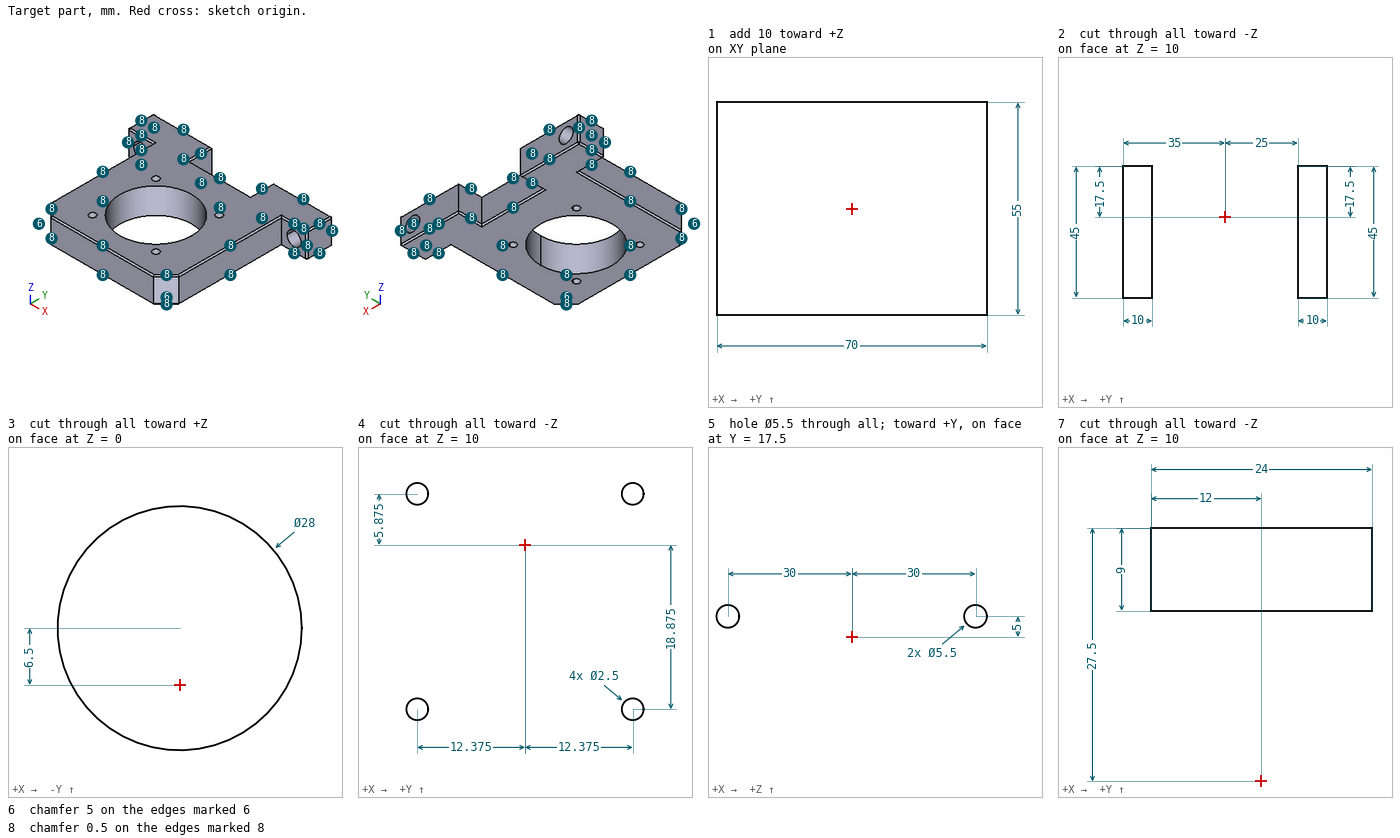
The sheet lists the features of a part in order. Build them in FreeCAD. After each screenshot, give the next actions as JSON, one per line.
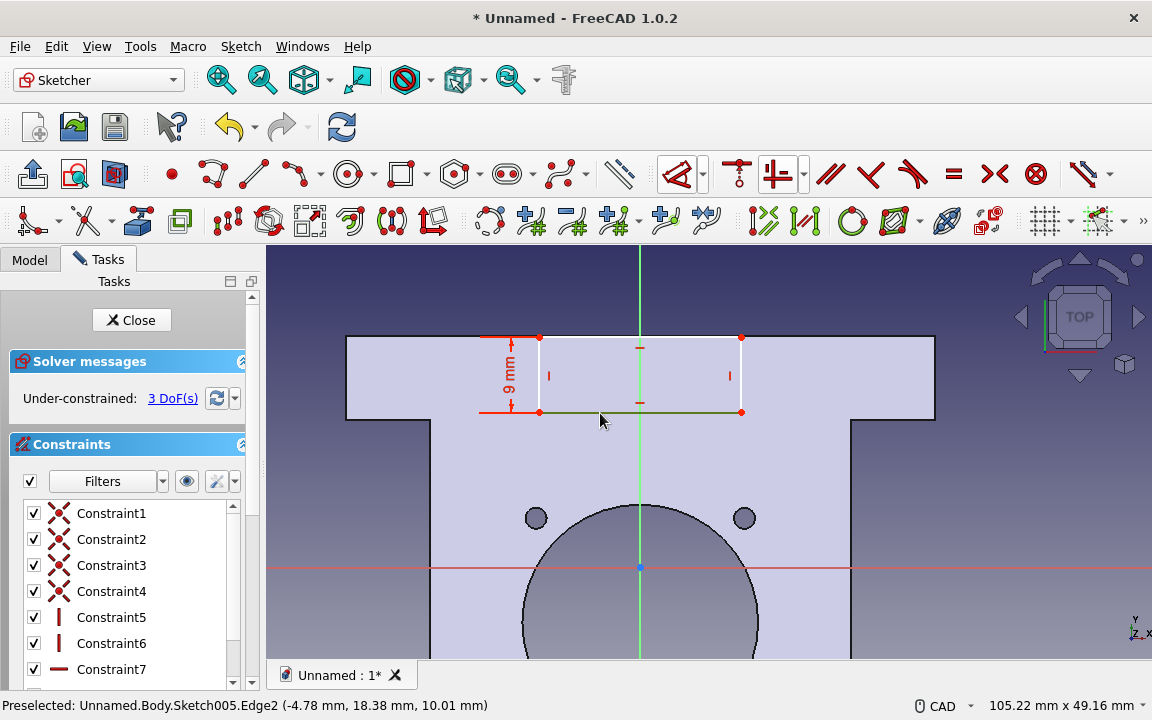
{"action": "key", "text": "l"}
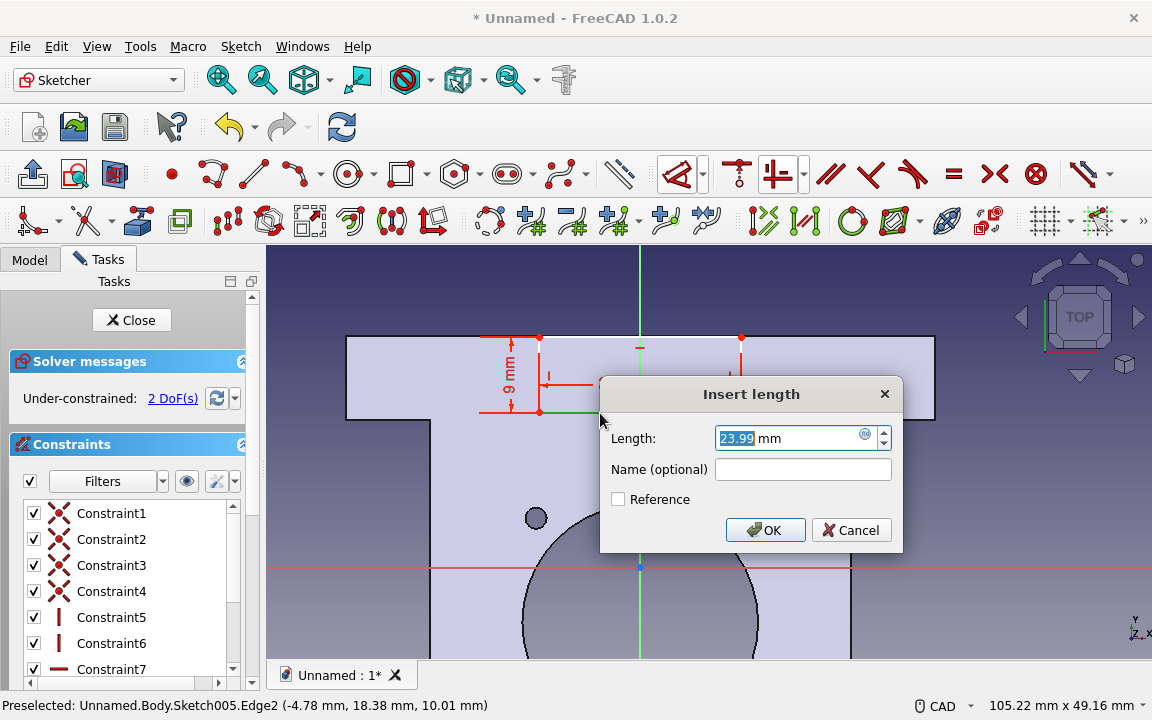
{"action": "type", "text": "24"}
{"action": "key", "text": "Return"}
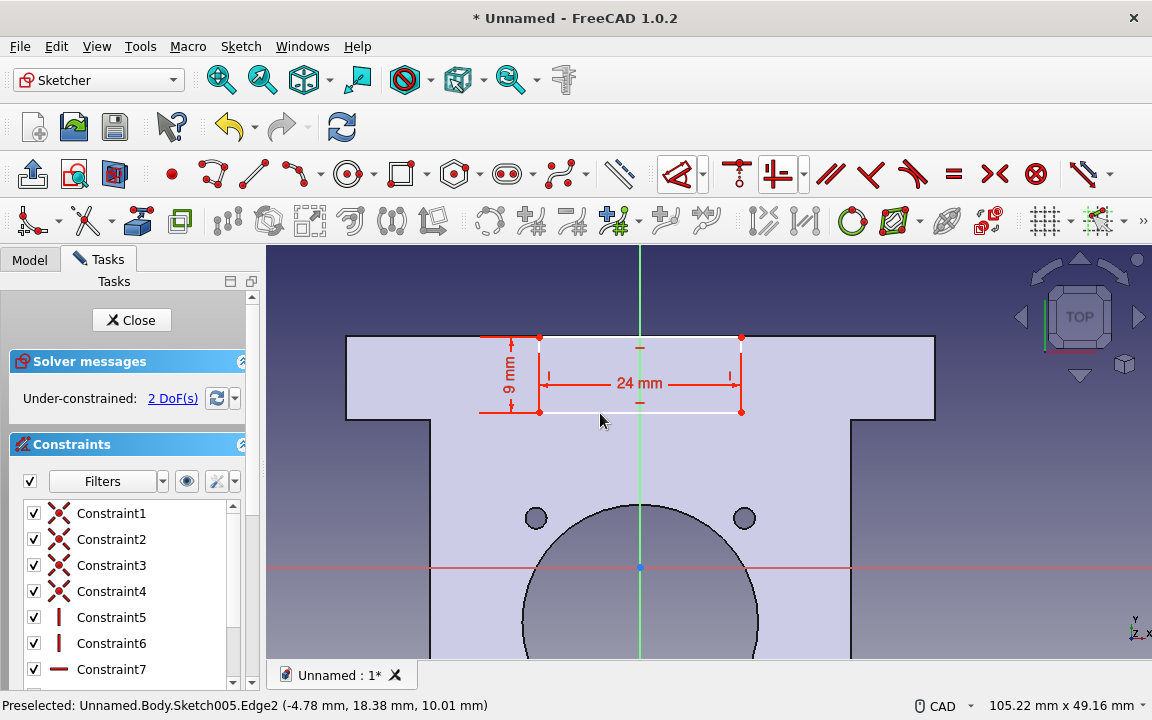
{"action": "left_click", "coordinate": [539, 337]}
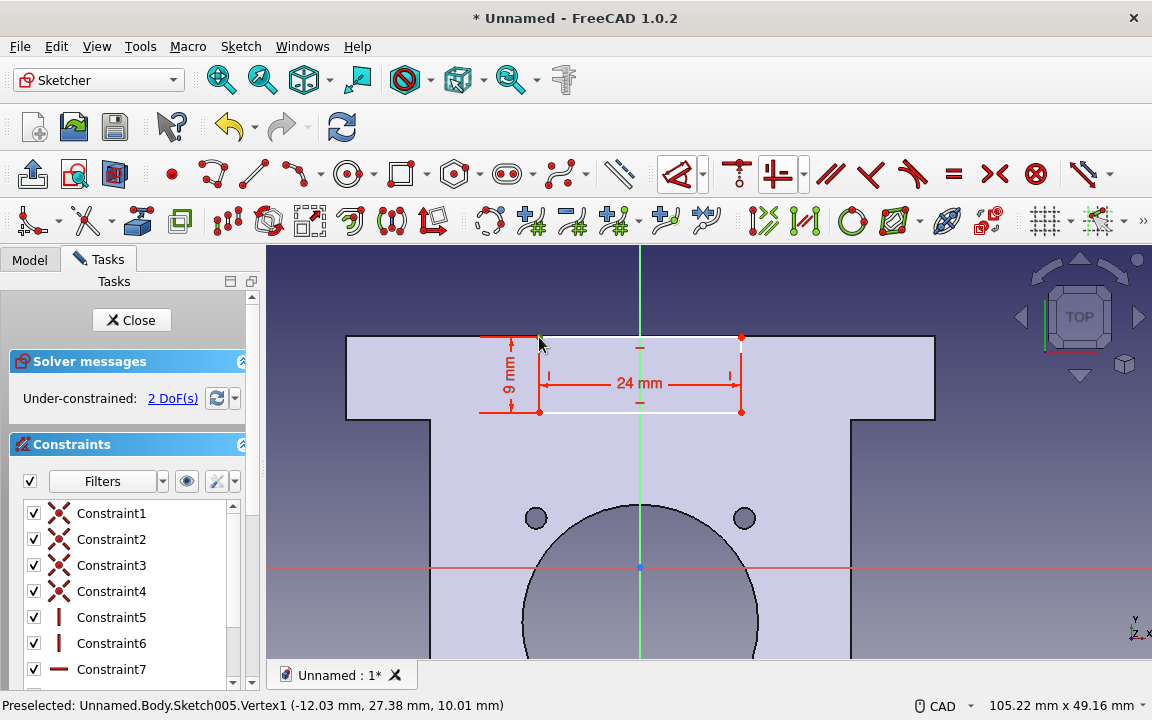
{"action": "left_click", "coordinate": [702, 174]}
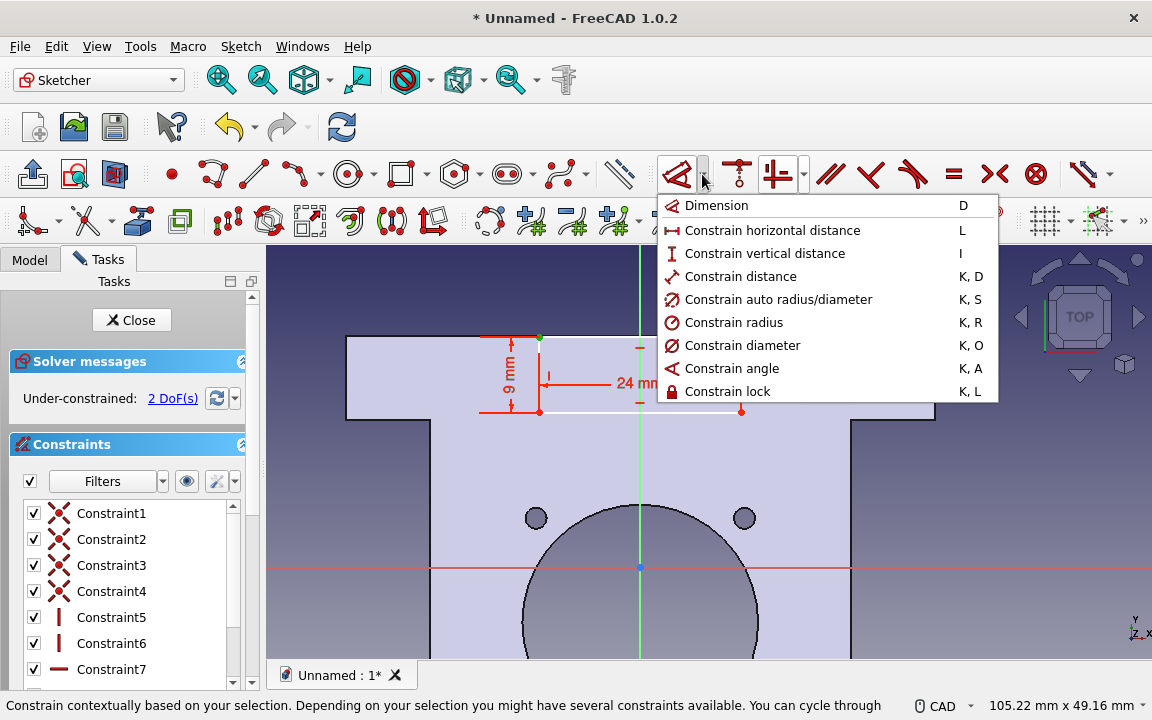
{"action": "left_click", "coordinate": [828, 230]}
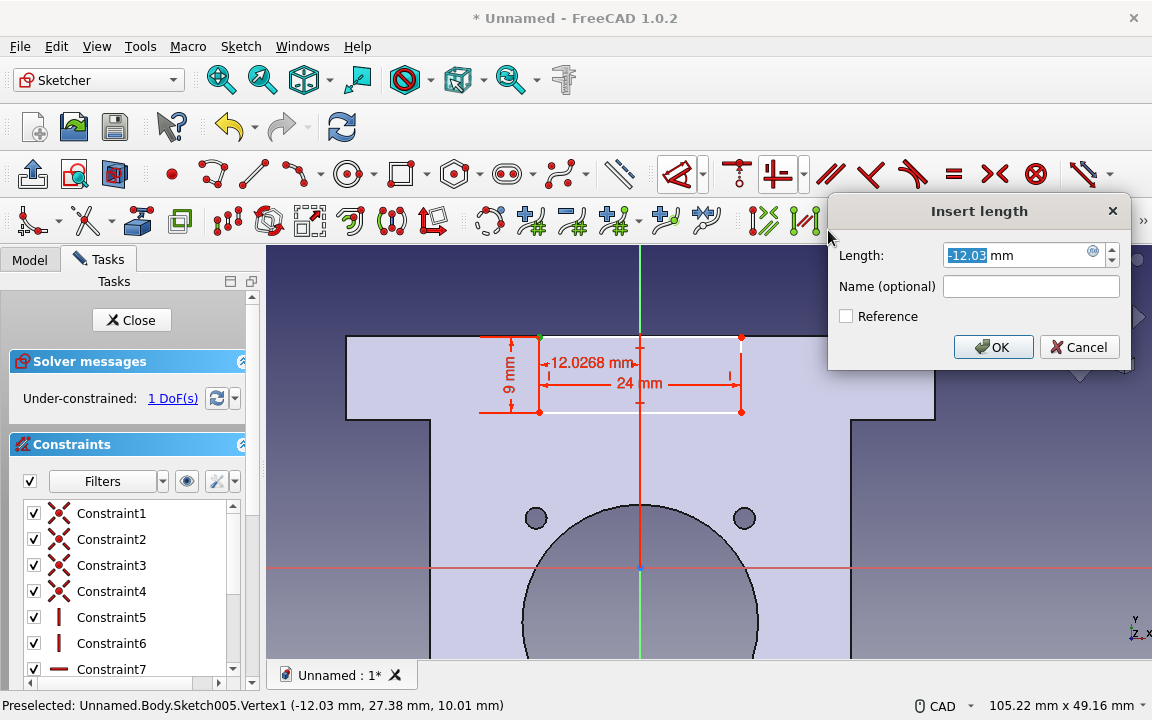
{"action": "type", "text": "-12"}
{"action": "key", "text": "Return"}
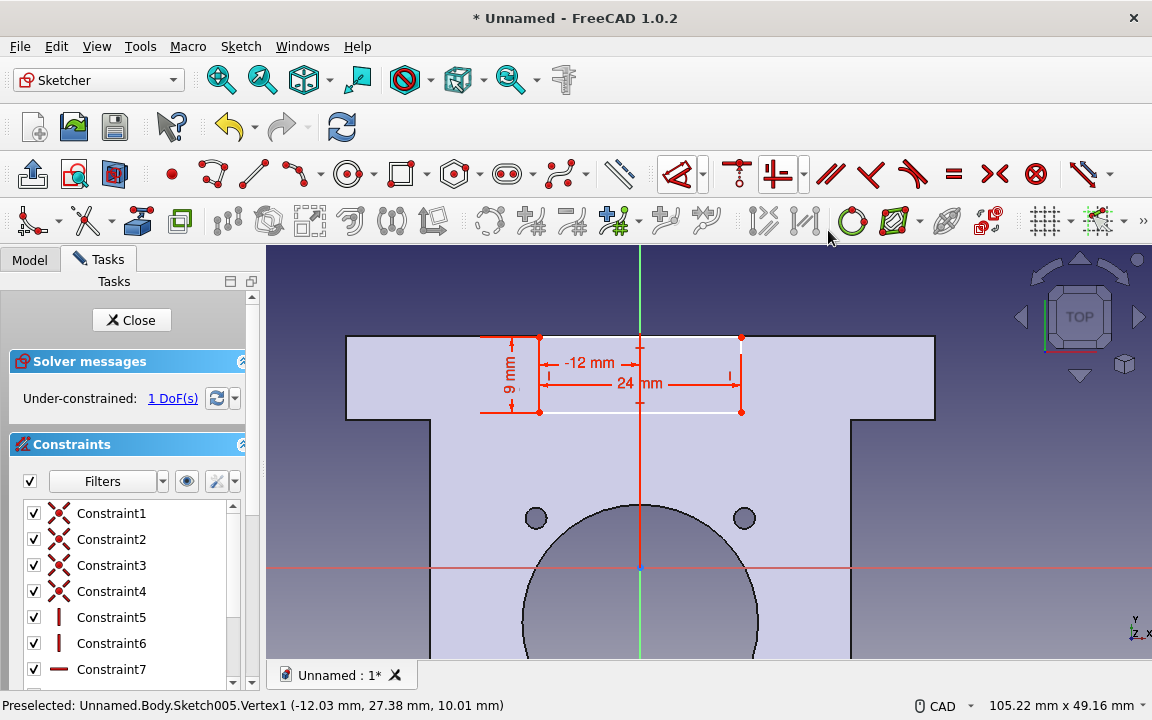
{"action": "left_click", "coordinate": [539, 337]}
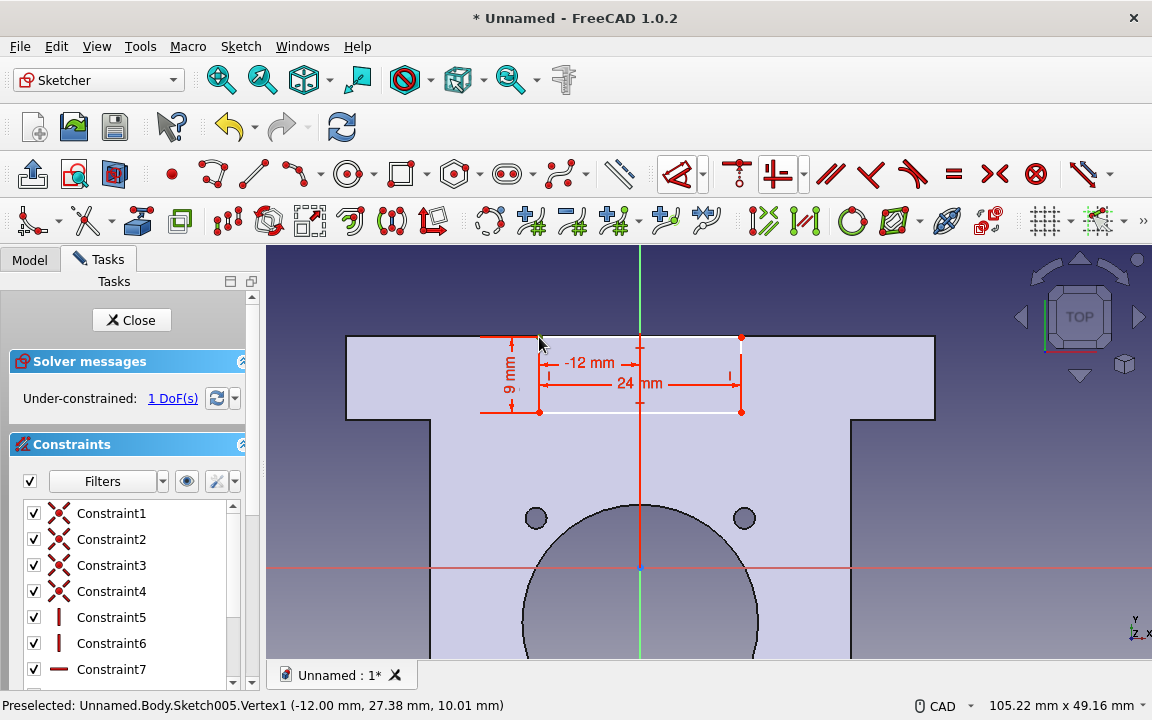
{"action": "left_click", "coordinate": [702, 174]}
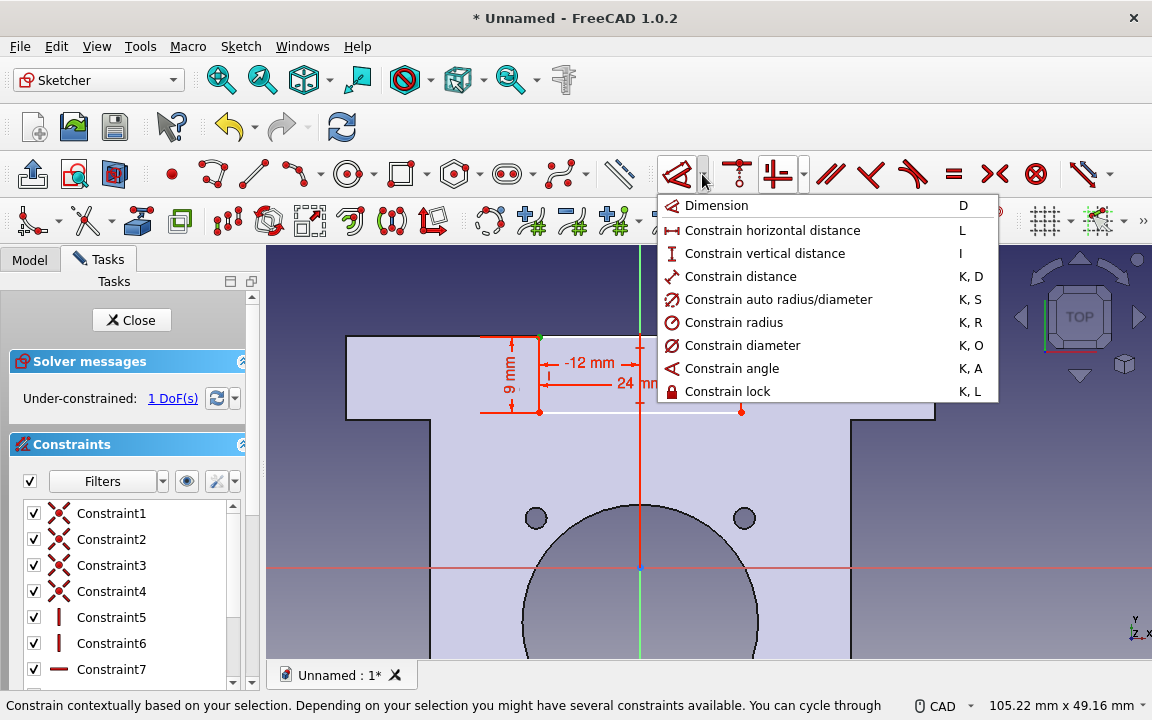
{"action": "left_click", "coordinate": [828, 254]}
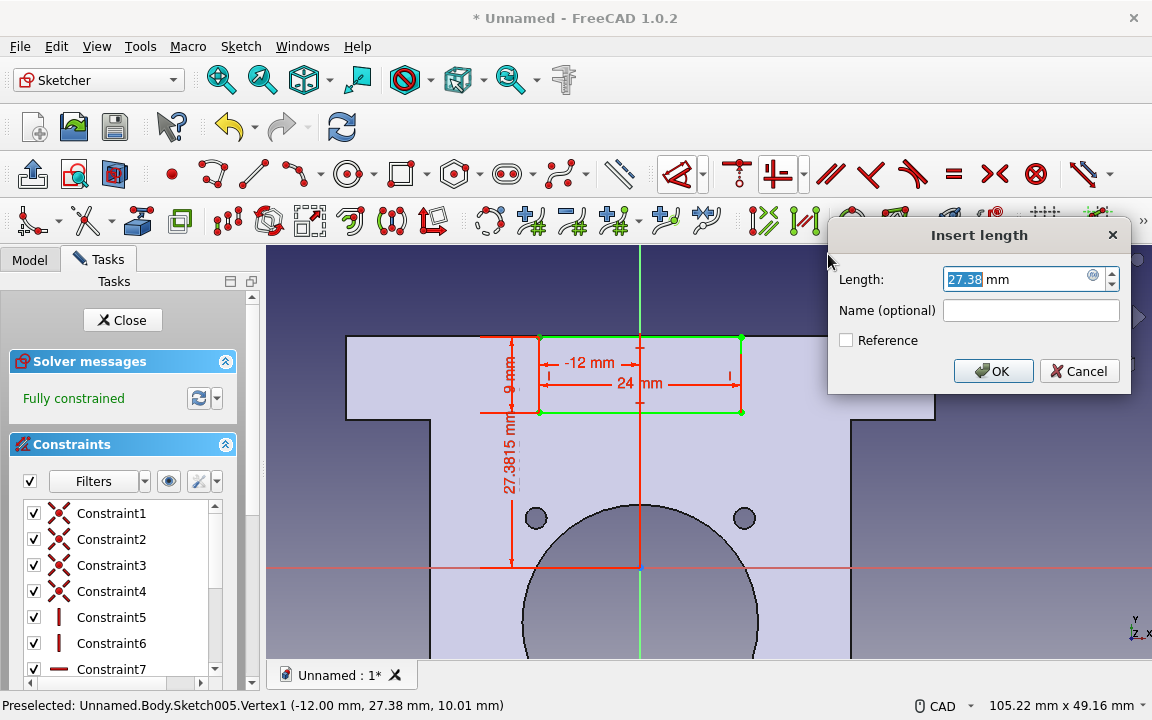
{"action": "type", "text": "27.5"}
{"action": "key", "text": "Return"}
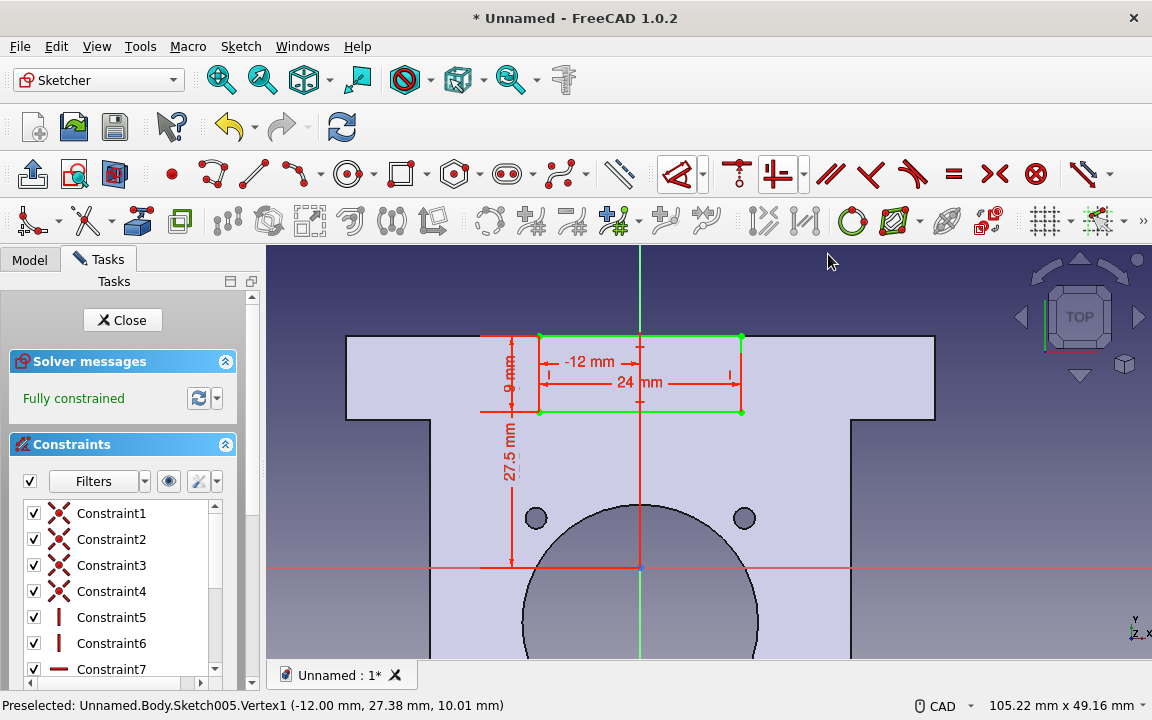
{"action": "left_click", "coordinate": [123, 320]}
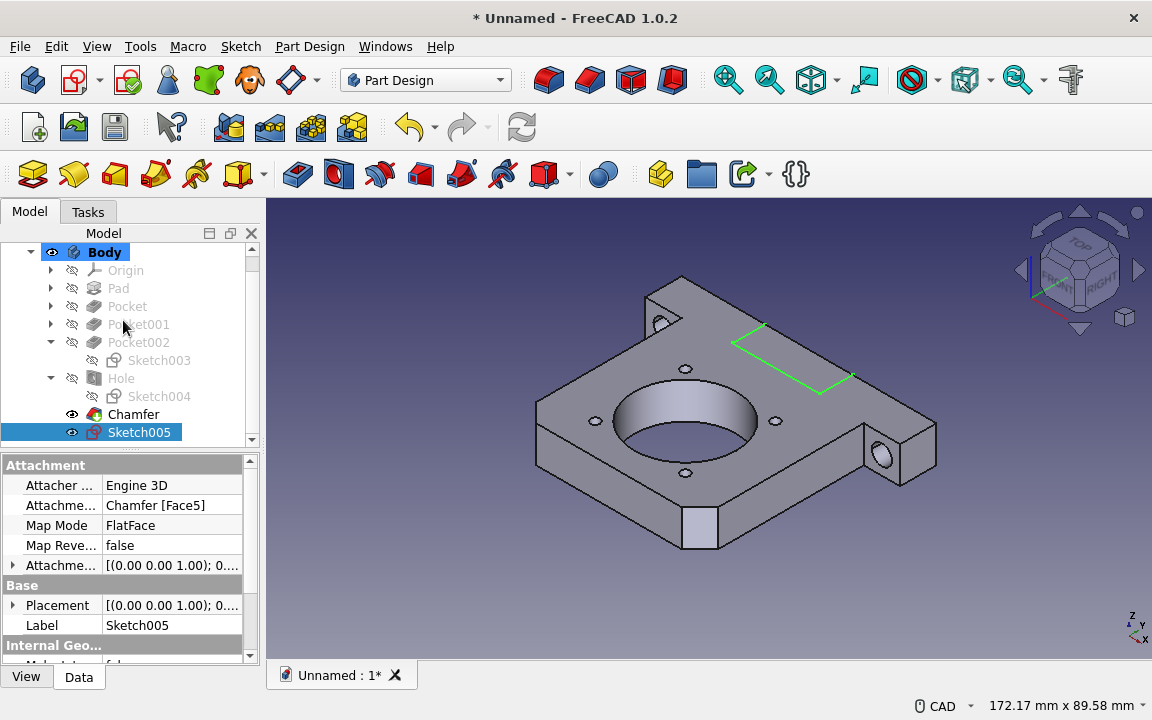
{"action": "left_click", "coordinate": [298, 174]}